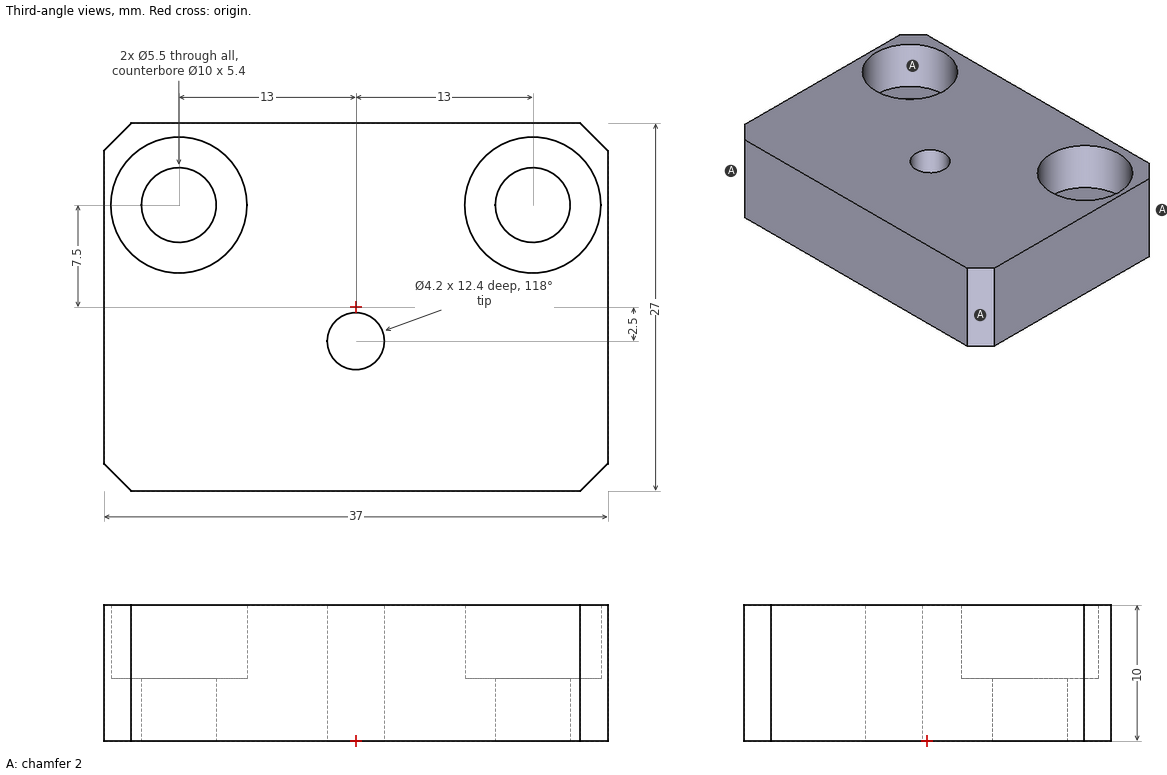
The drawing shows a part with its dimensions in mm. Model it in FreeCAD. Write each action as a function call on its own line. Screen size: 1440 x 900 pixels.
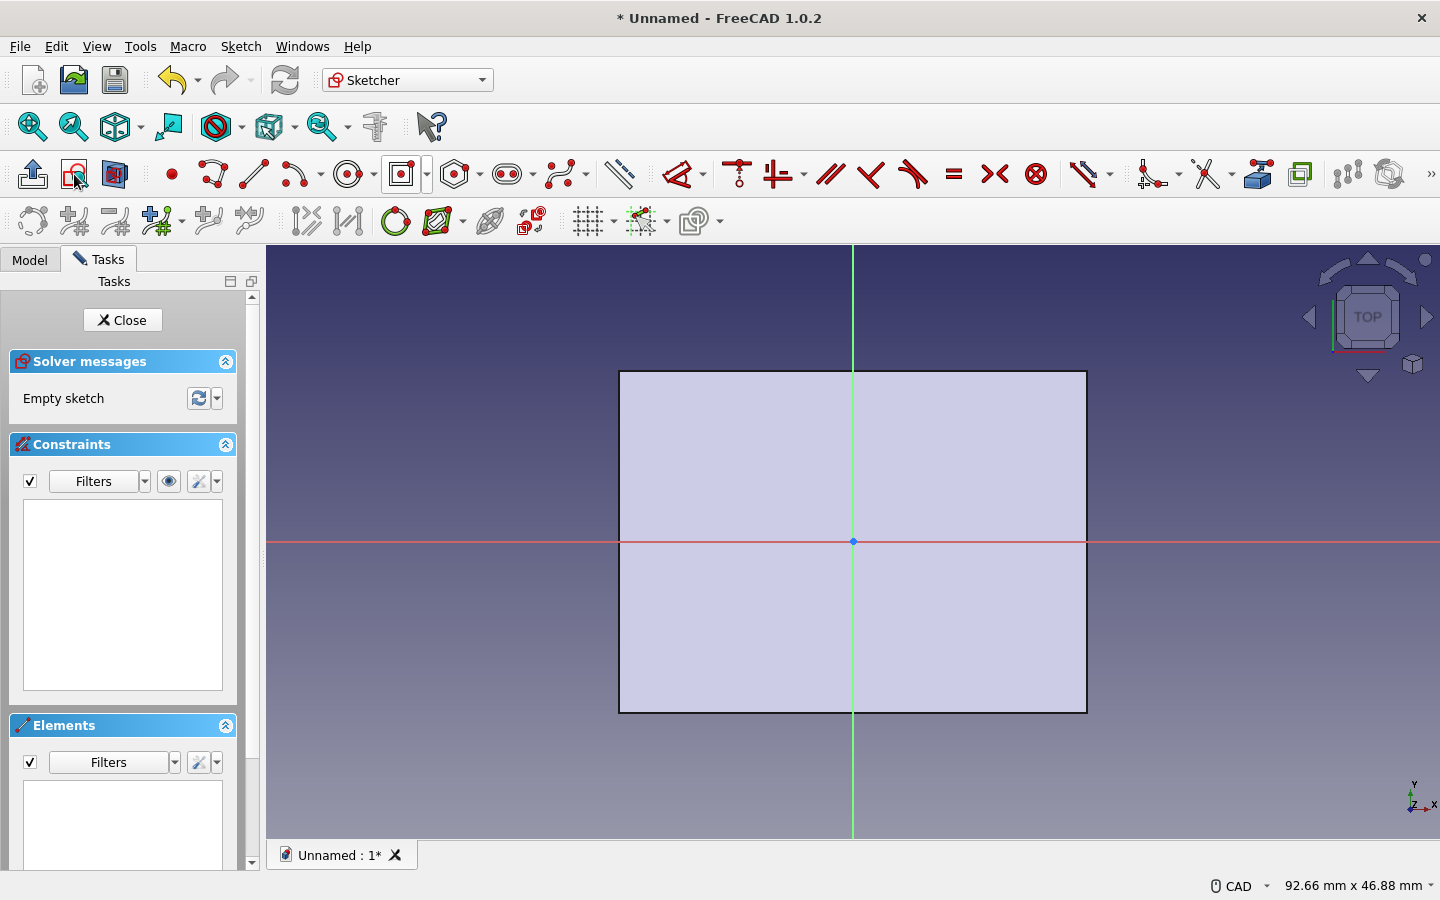
scroll(936, 398, up, 3)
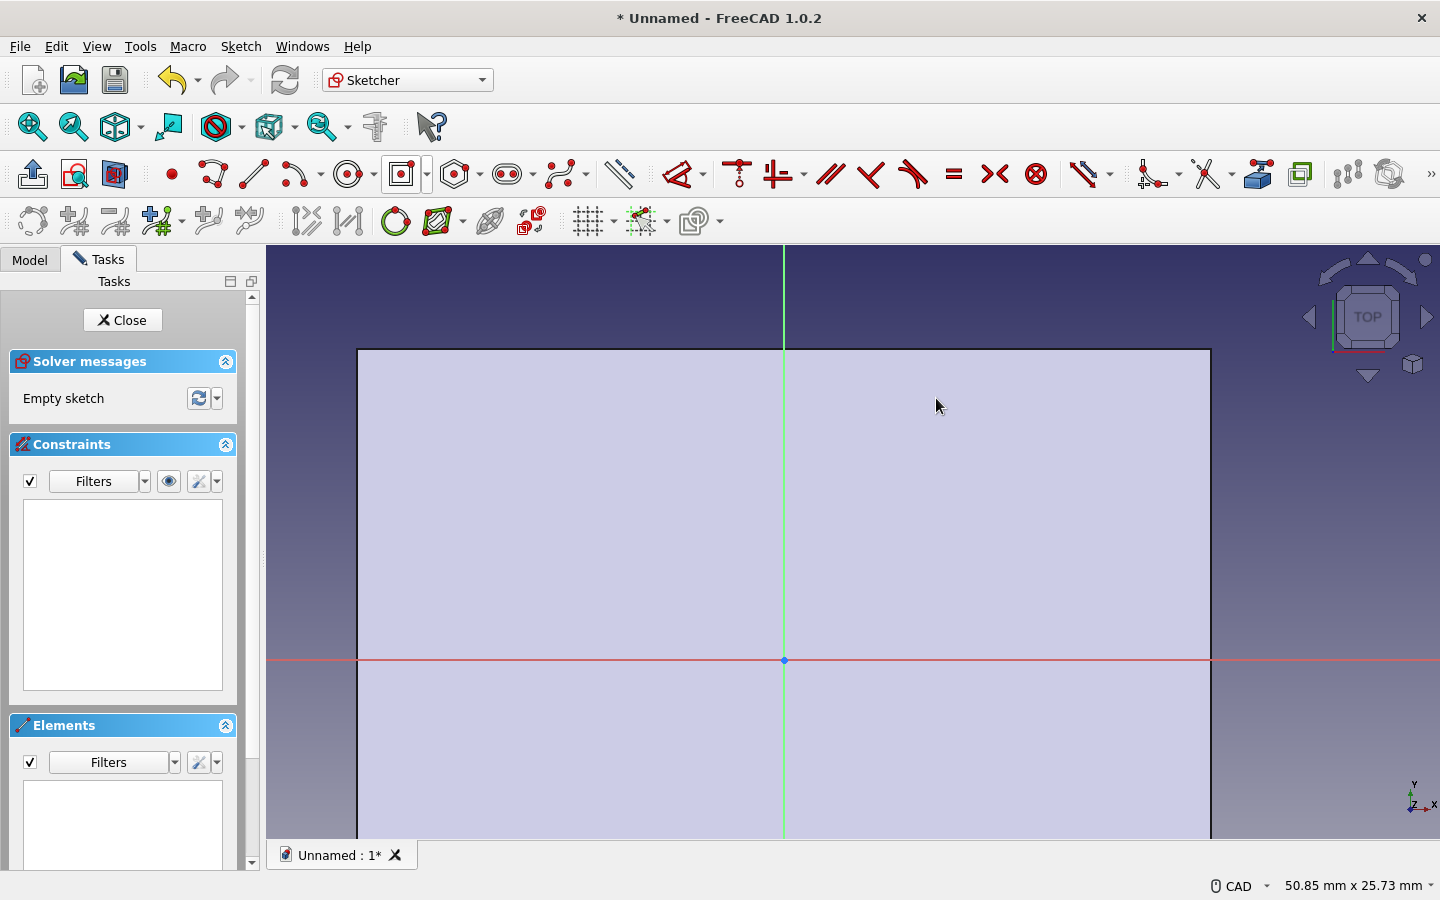
click(348, 174)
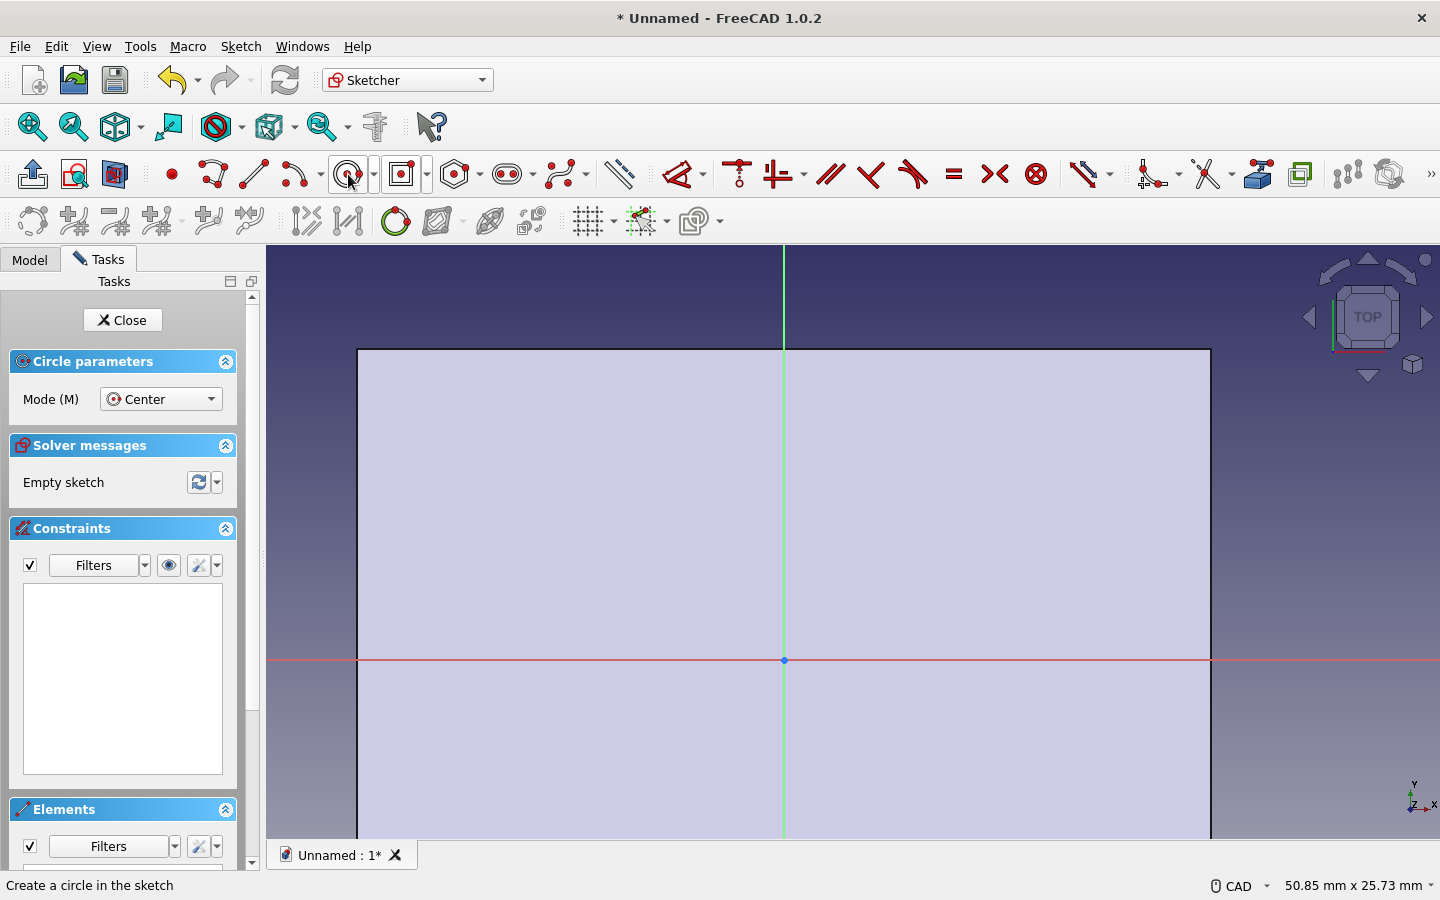
click(484, 487)
move(529, 442)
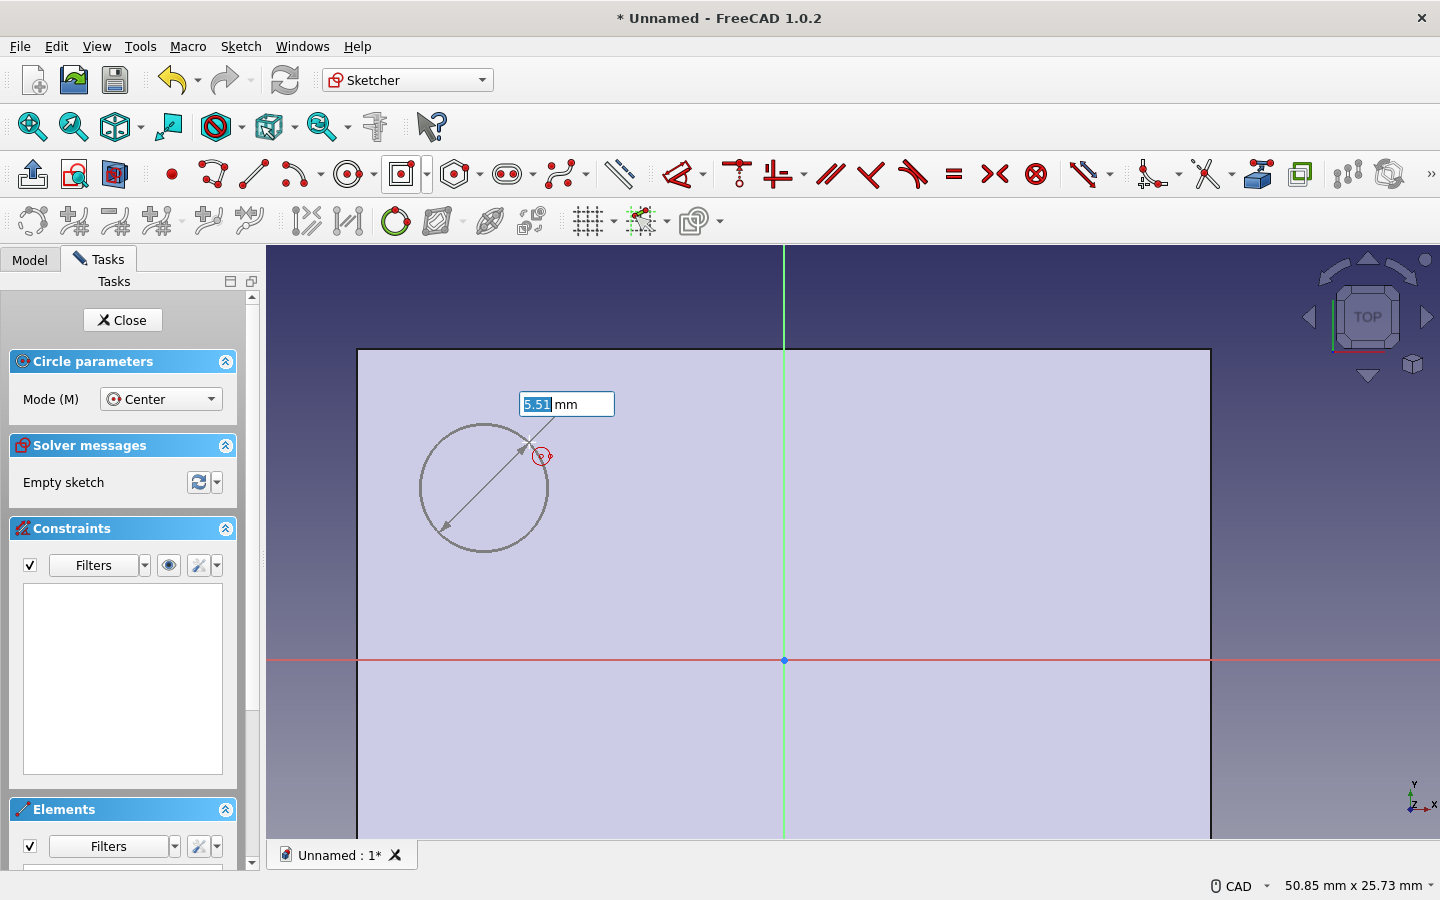
text(5.5)
key(Return)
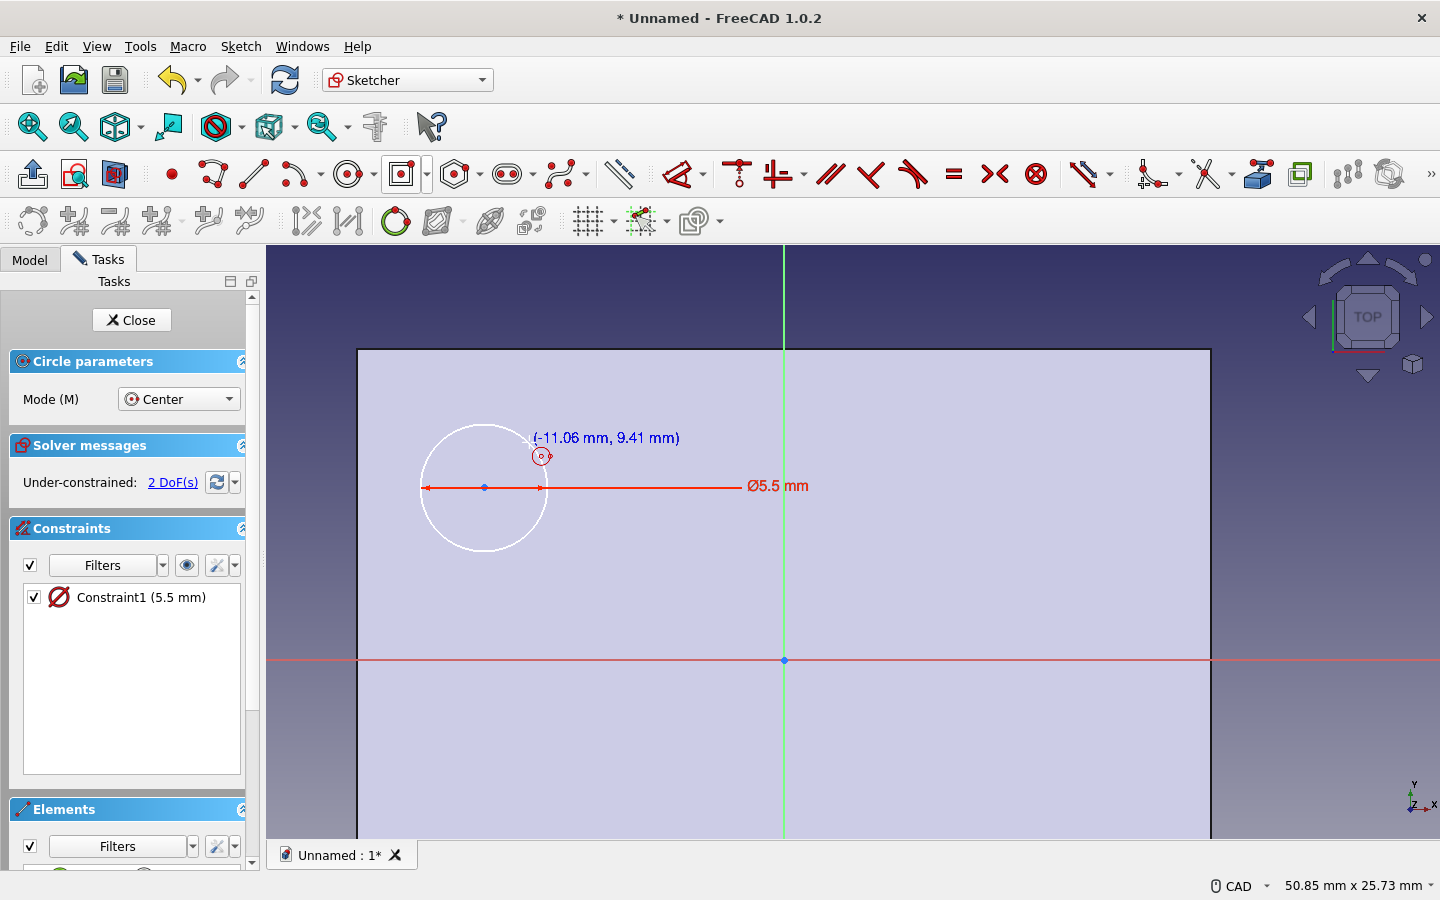
click(1084, 487)
move(1129, 442)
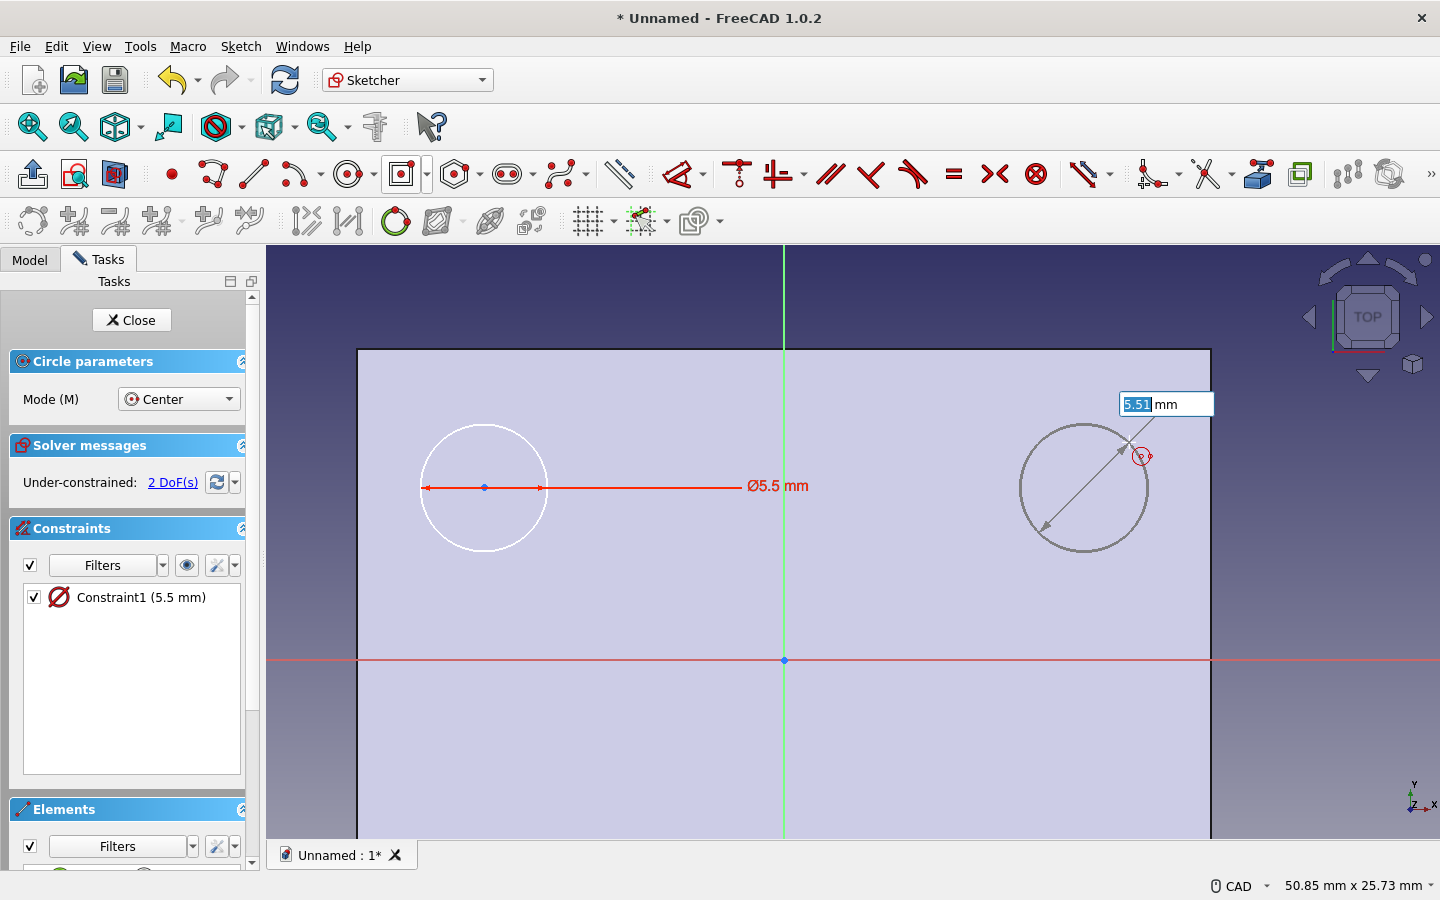
text(5.5)
key(Return)
key(Escape)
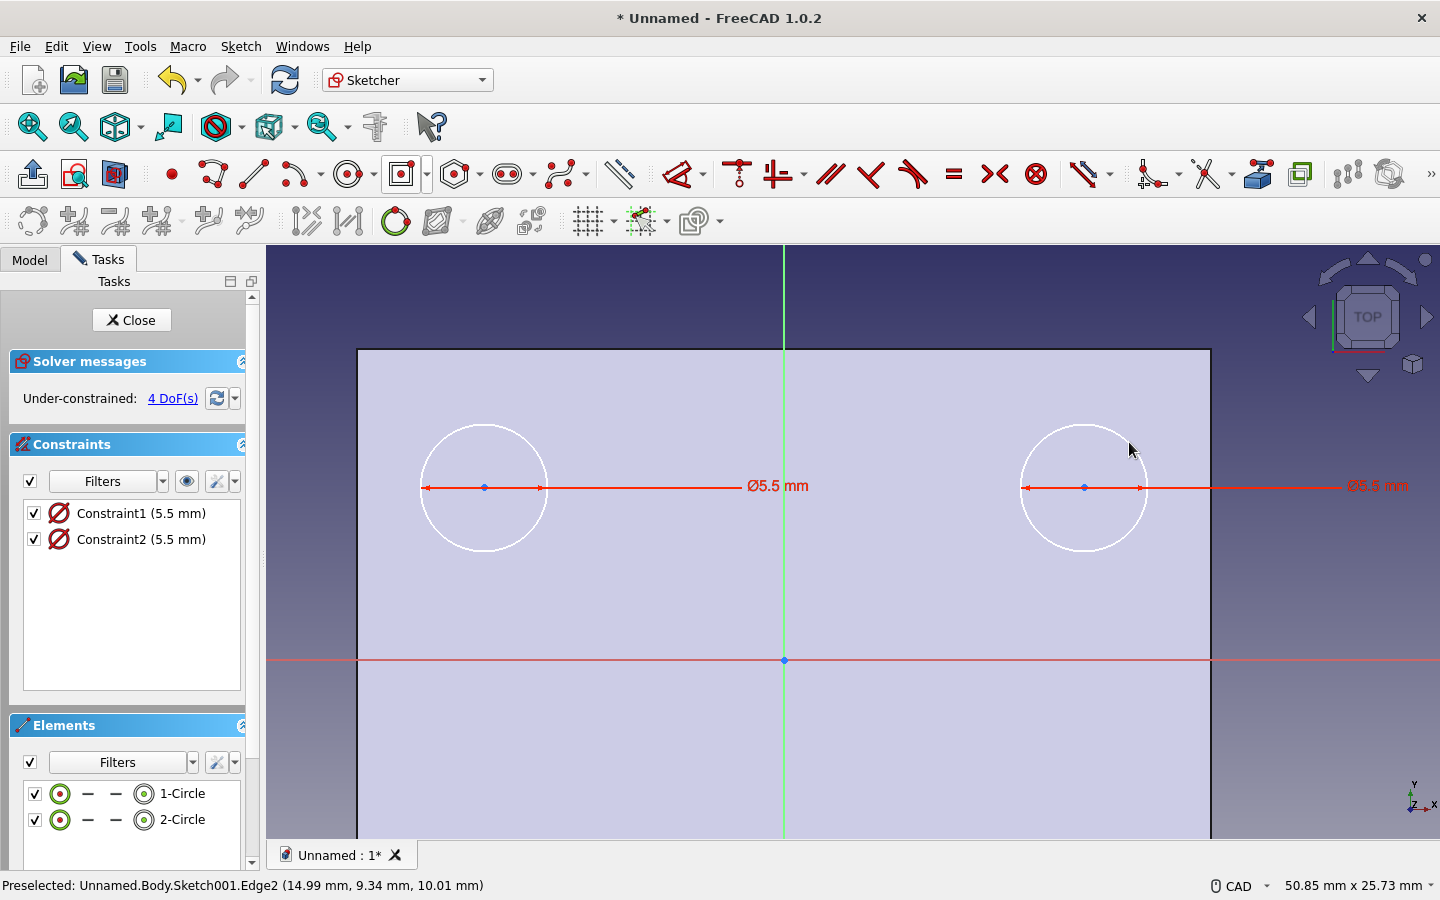
click(484, 488)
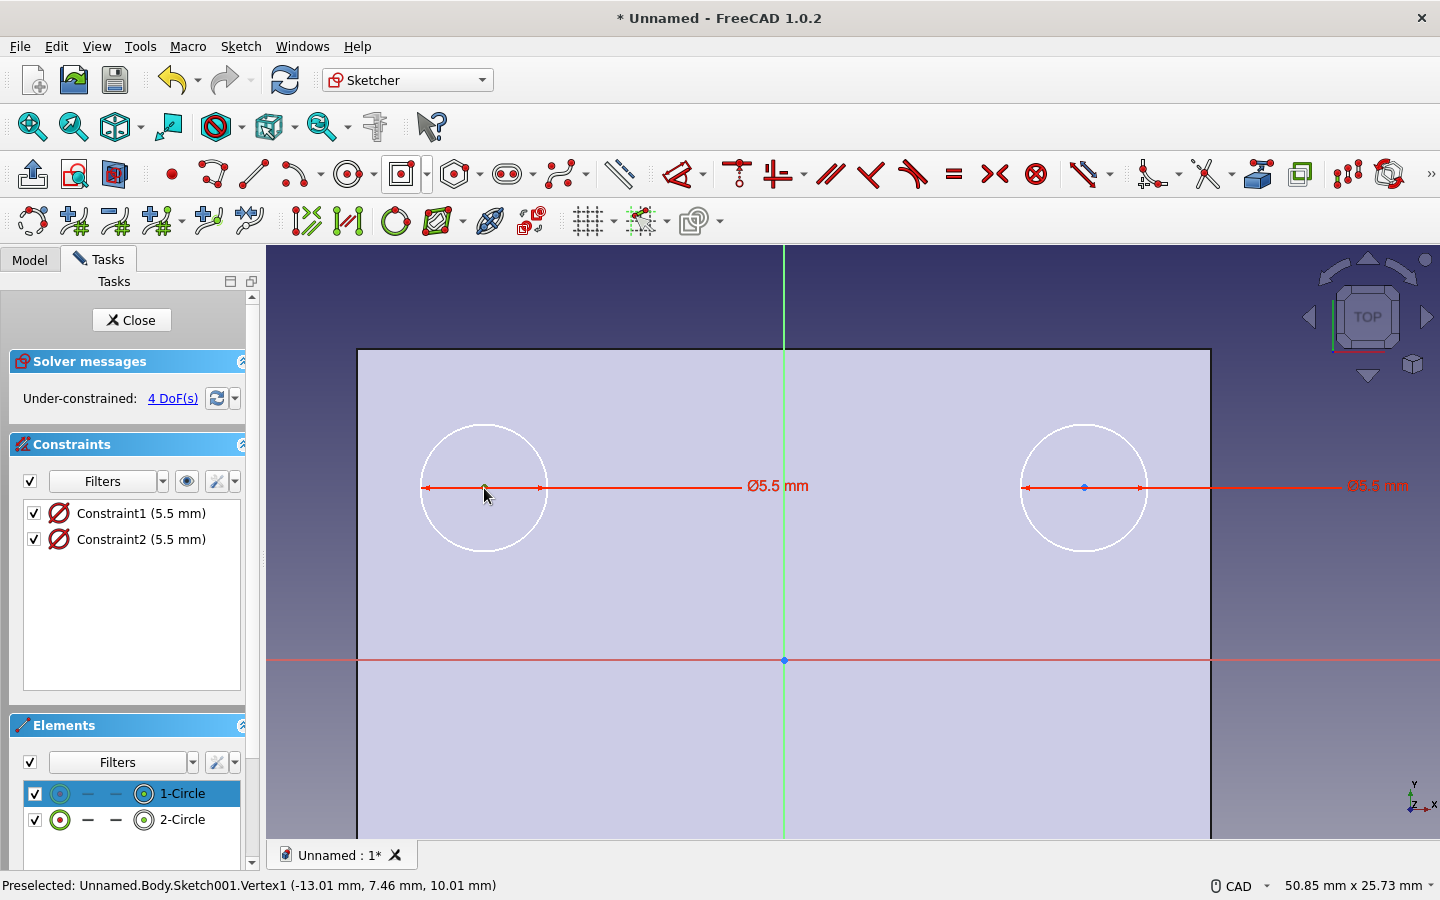
click(1084, 488)